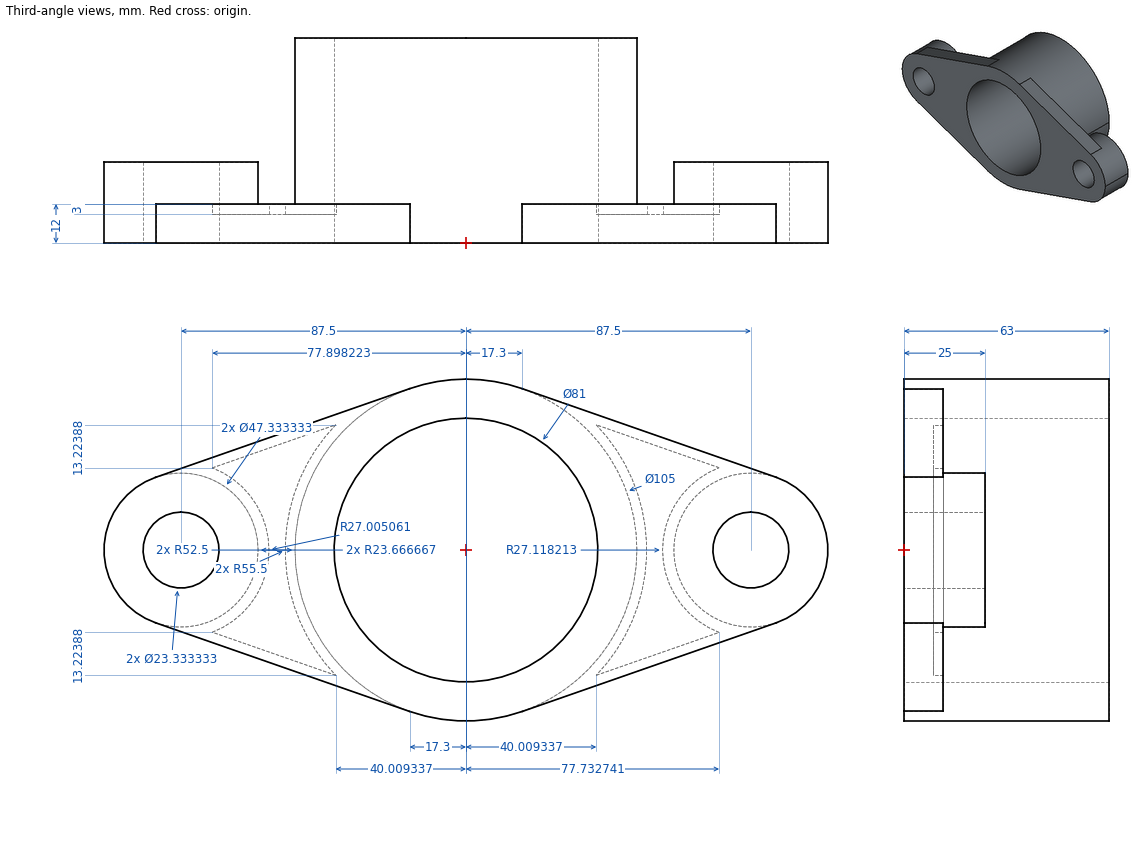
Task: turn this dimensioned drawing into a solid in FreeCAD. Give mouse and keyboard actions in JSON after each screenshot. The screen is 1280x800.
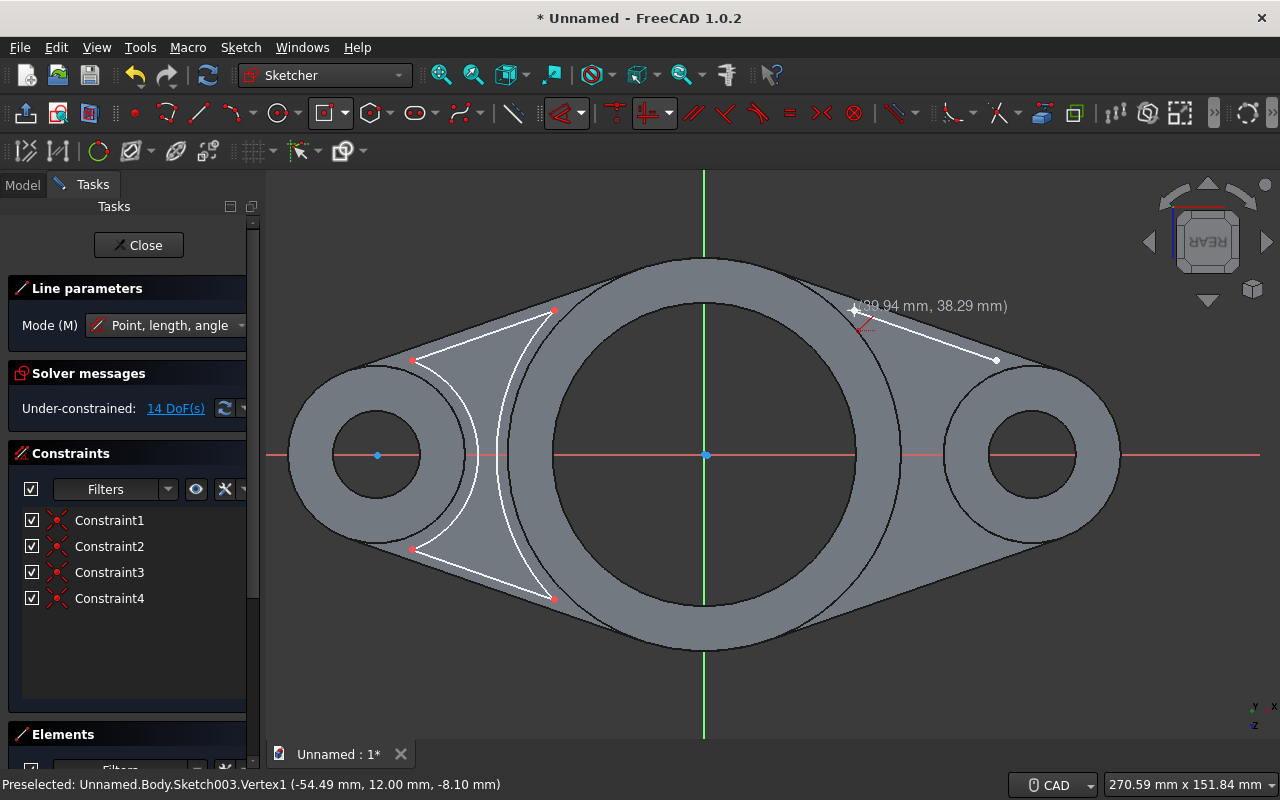
{"action": "left_click", "coordinate": [854, 599]}
{"action": "left_click", "coordinate": [996, 549]}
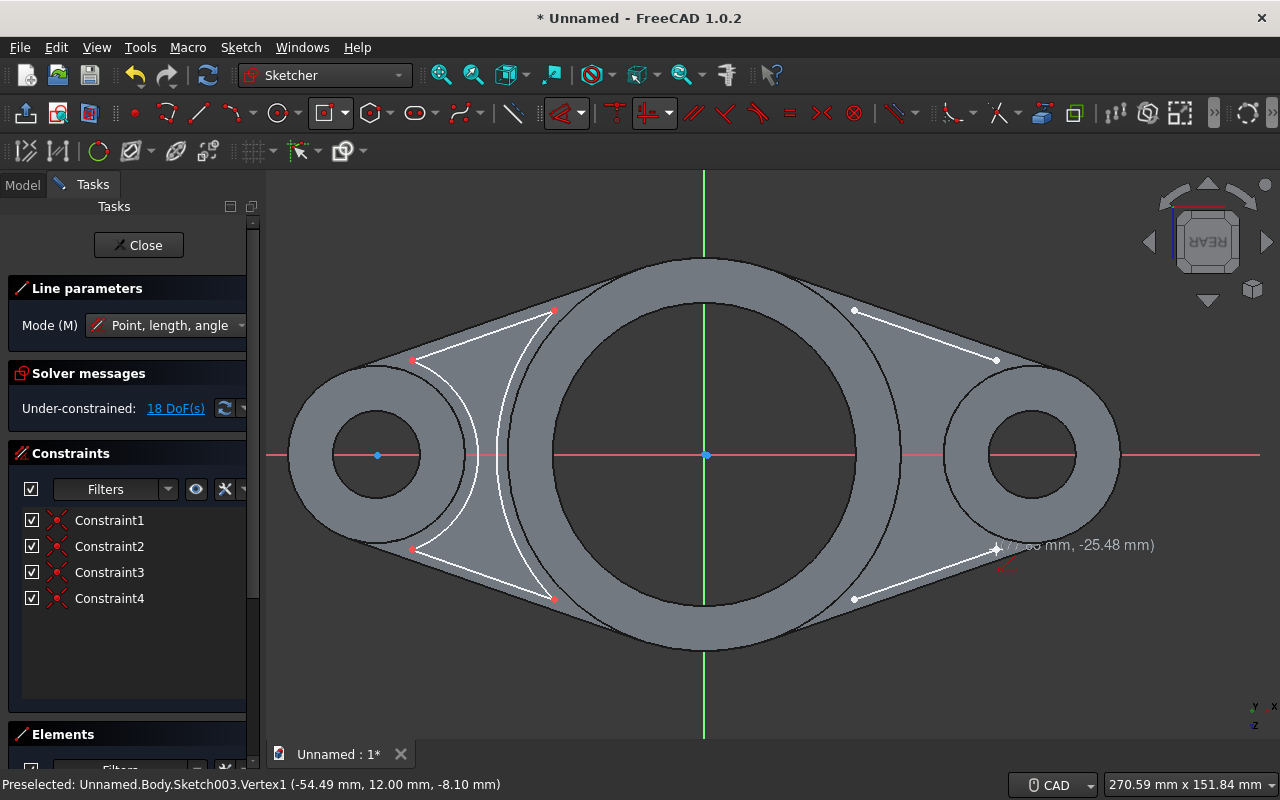
{"action": "left_click", "coordinate": [232, 114]}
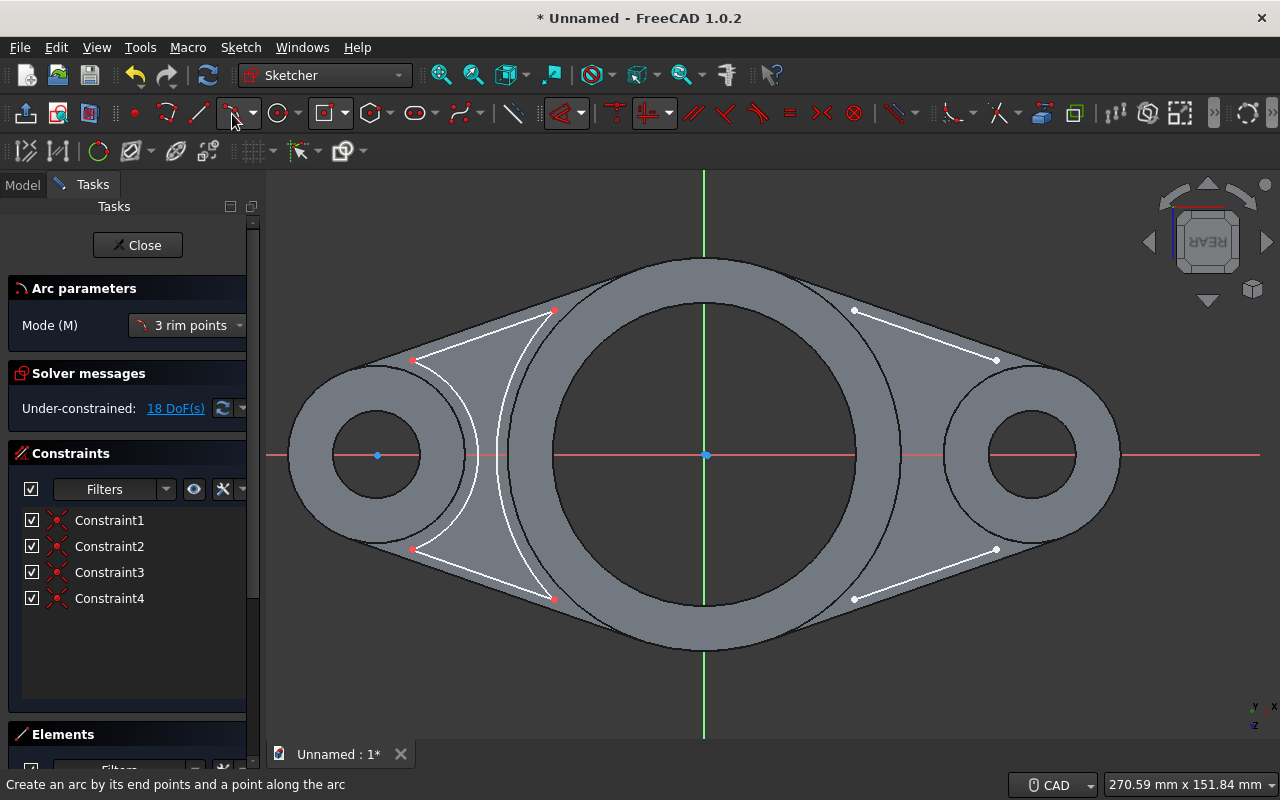
{"action": "left_click", "coordinate": [854, 311]}
{"action": "left_click", "coordinate": [854, 600]}
{"action": "left_click", "coordinate": [910, 486]}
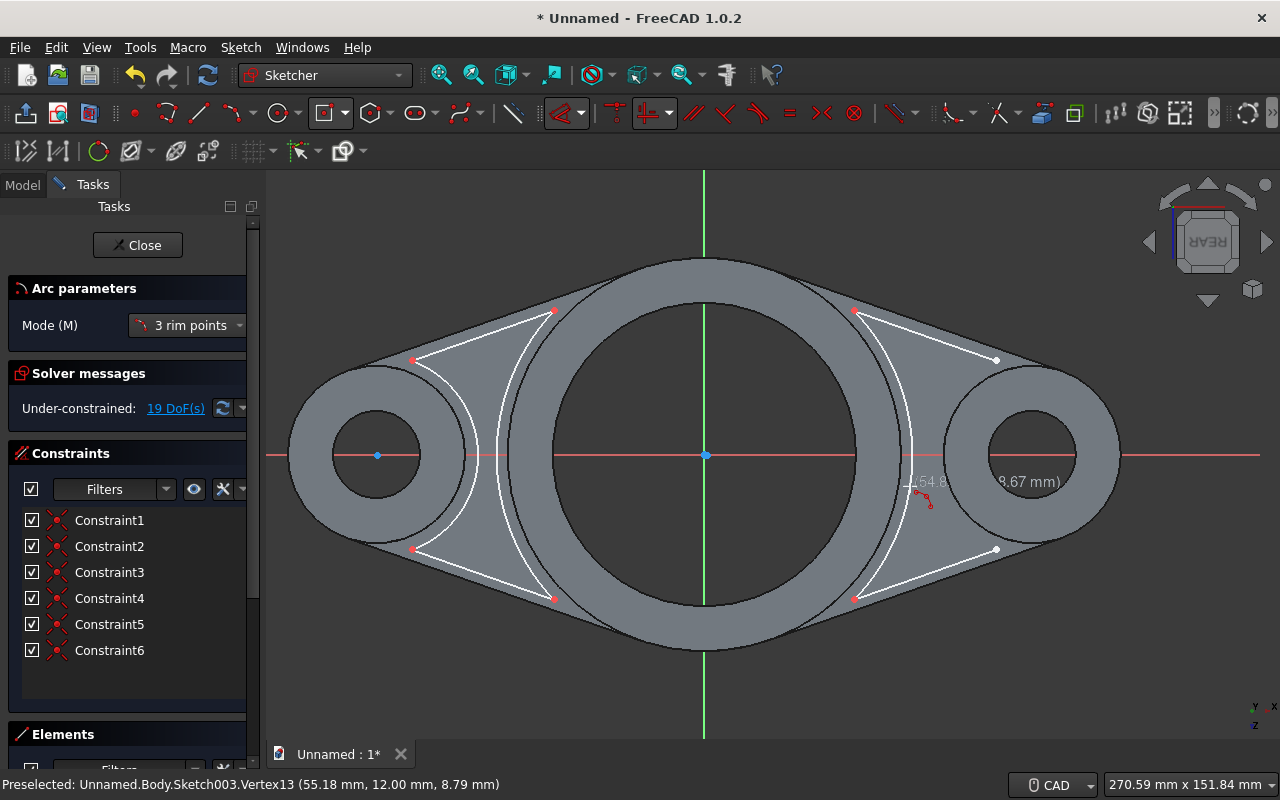
{"action": "left_click", "coordinate": [996, 550]}
{"action": "left_click", "coordinate": [996, 361]}
{"action": "left_click", "coordinate": [934, 430]}
{"action": "key", "text": "Escape"}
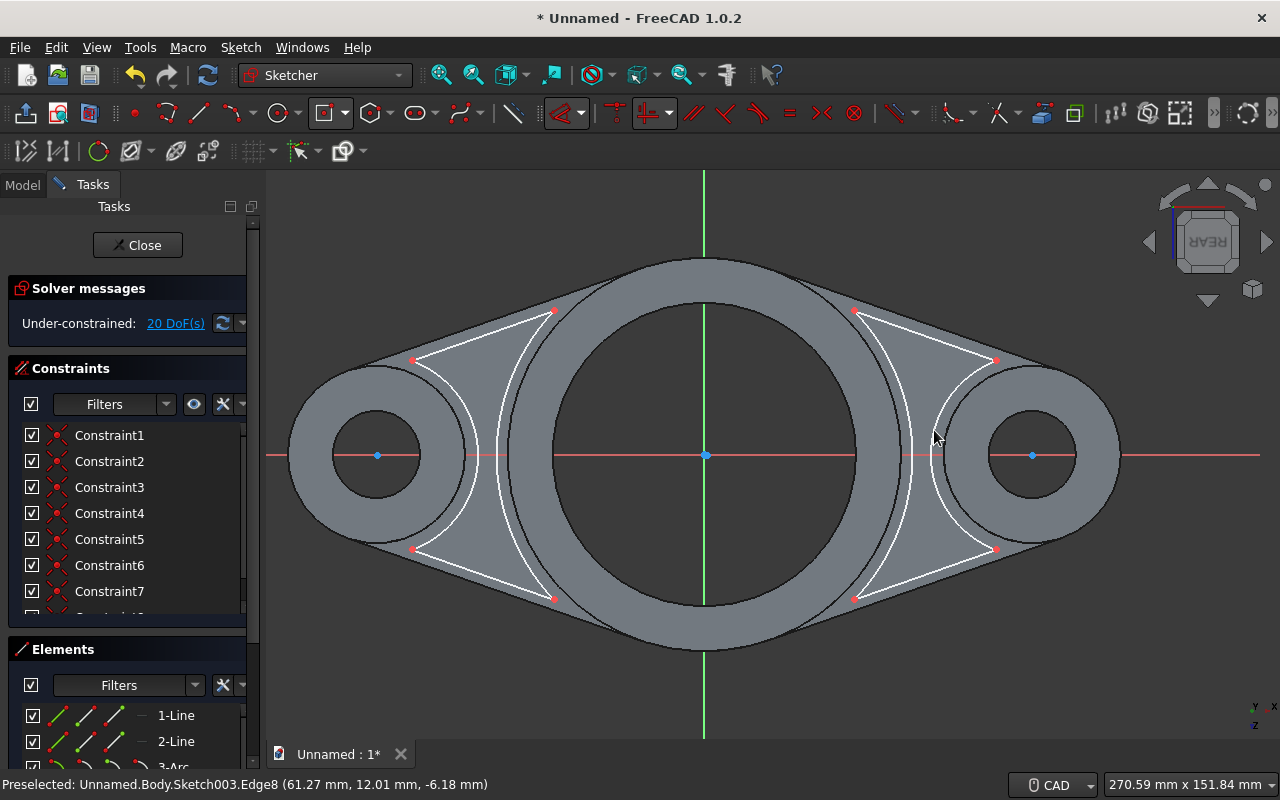
{"action": "left_click", "coordinate": [506, 393]}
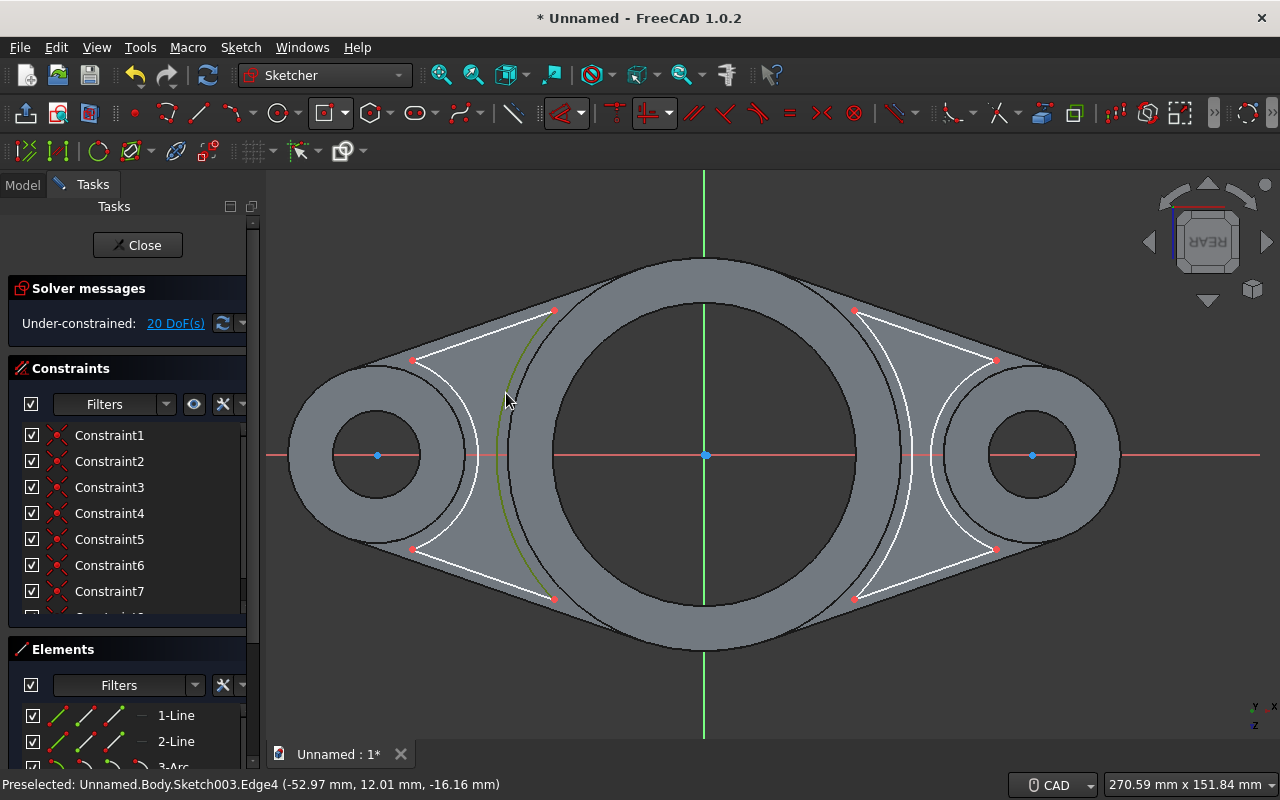
{"action": "left_click", "coordinate": [903, 518]}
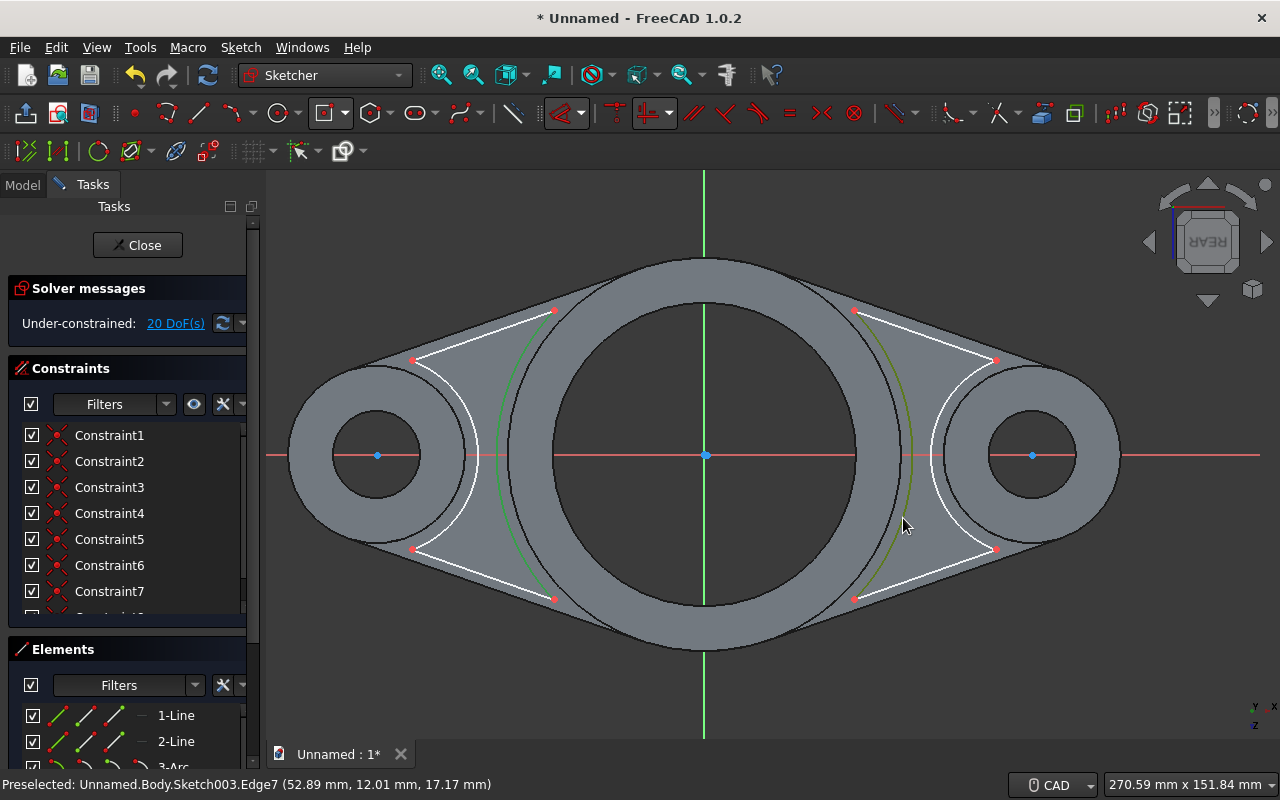
{"action": "left_click", "coordinate": [616, 114]}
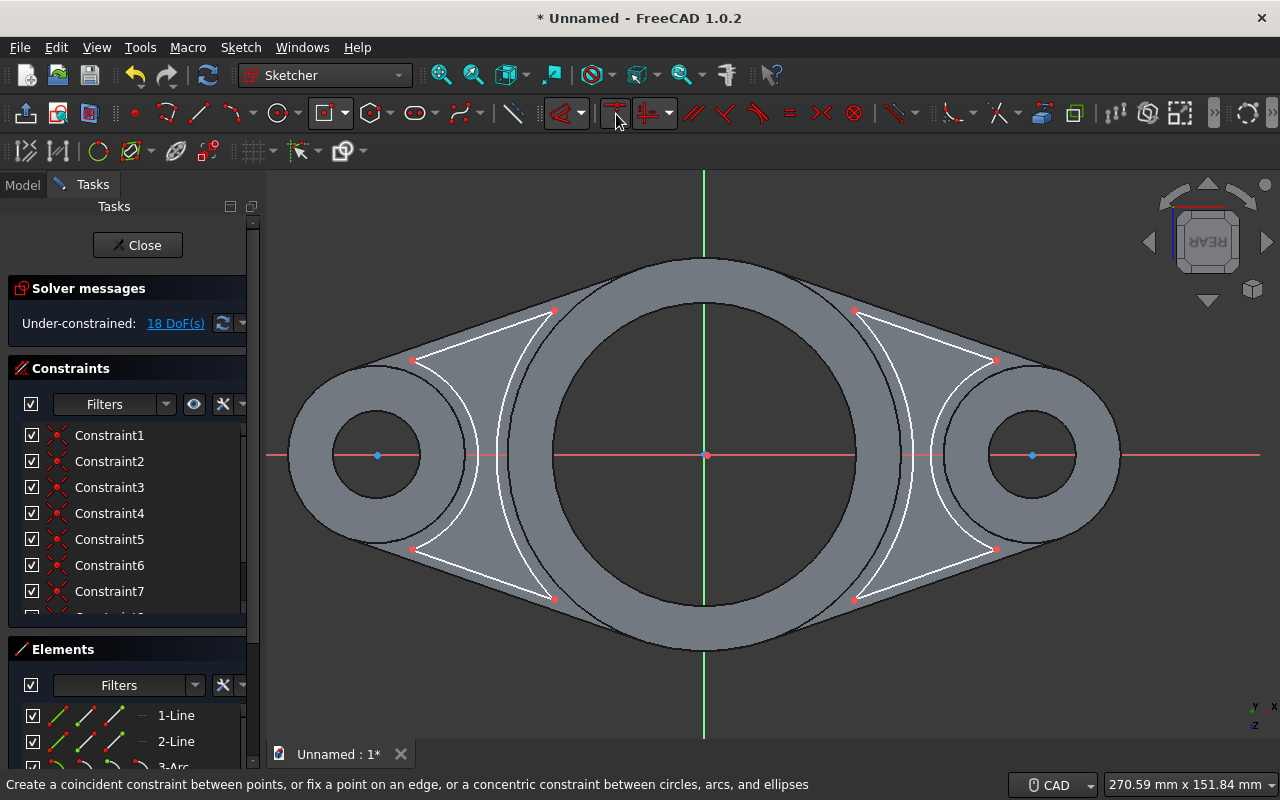
{"action": "left_click_drag", "start_coordinate": [694, 444], "coordinate": [717, 465]}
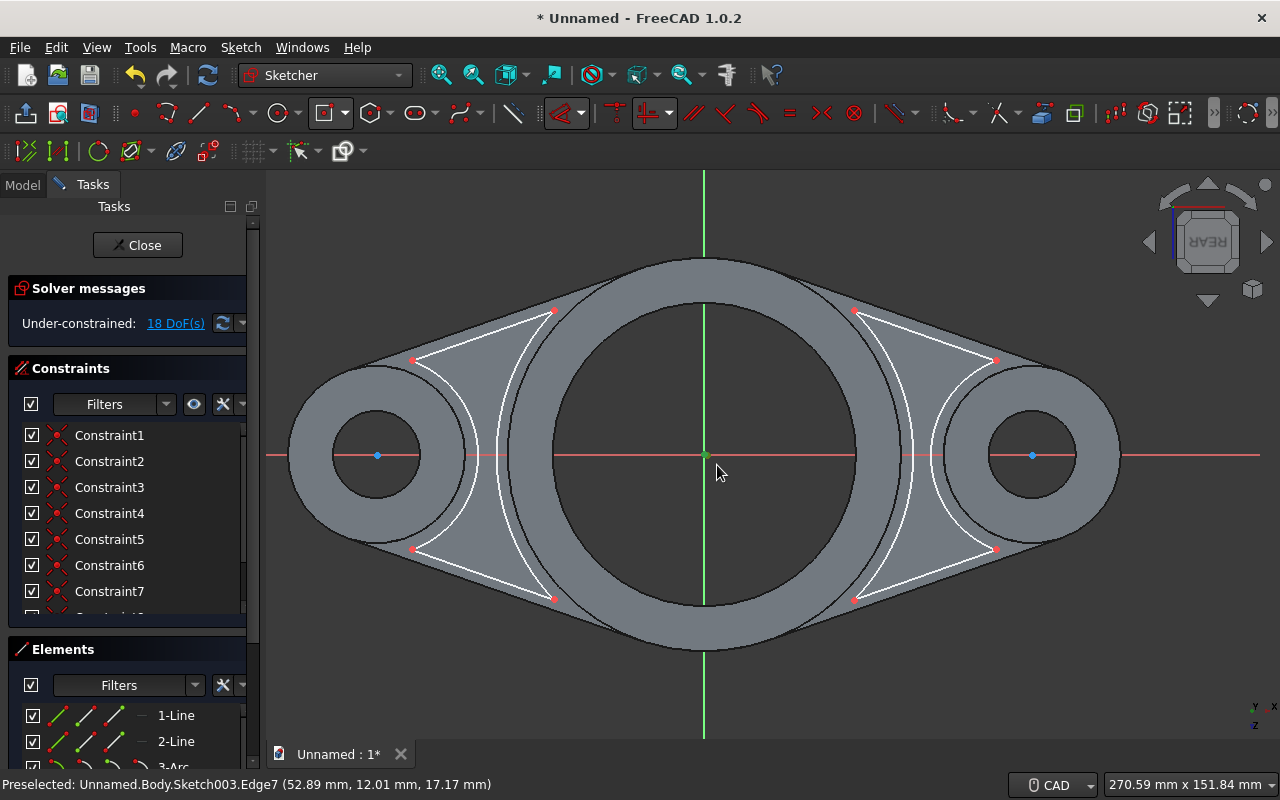
{"action": "key", "text": "c"}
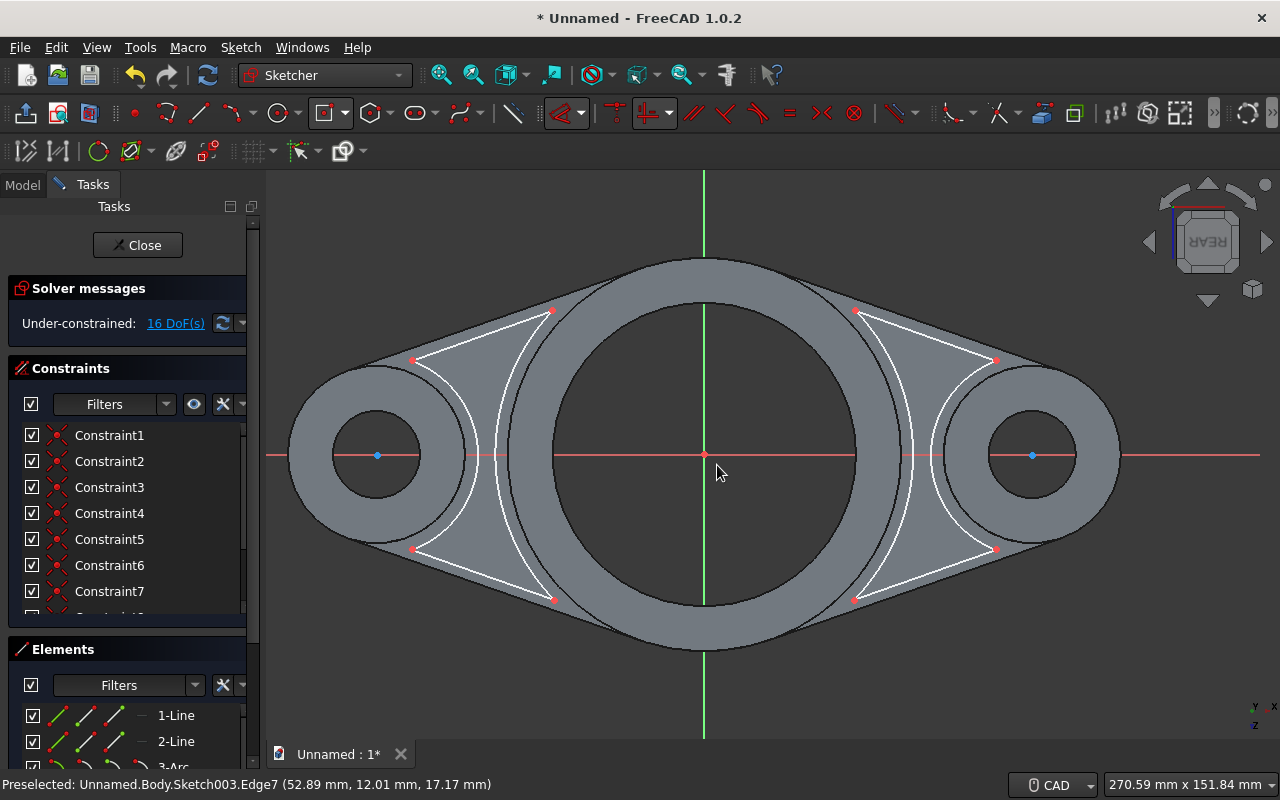
{"action": "left_click", "coordinate": [505, 393]}